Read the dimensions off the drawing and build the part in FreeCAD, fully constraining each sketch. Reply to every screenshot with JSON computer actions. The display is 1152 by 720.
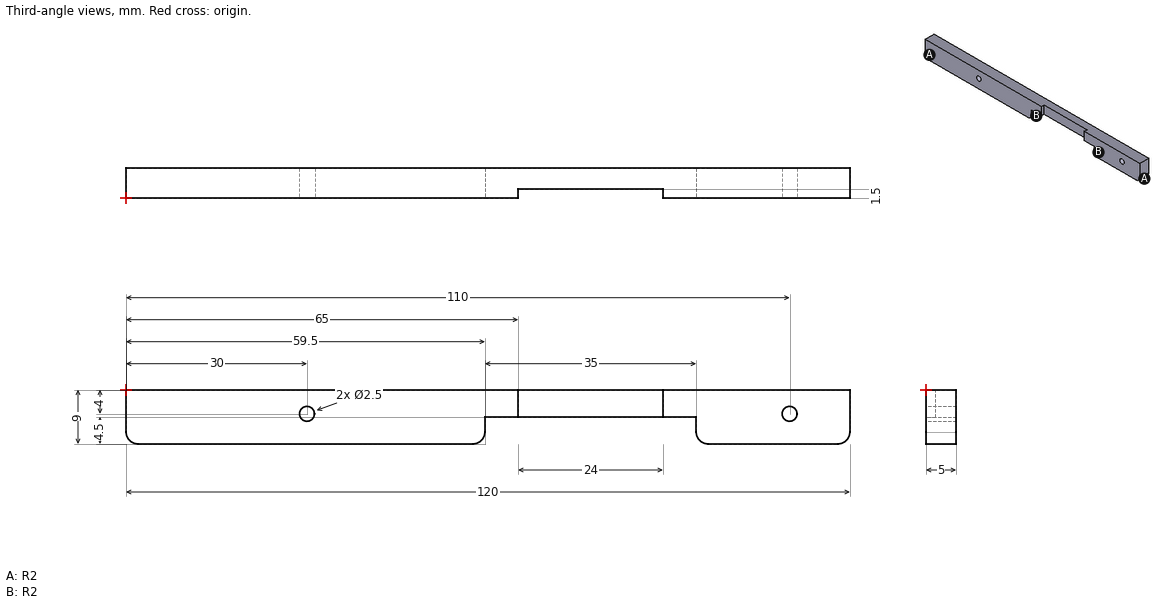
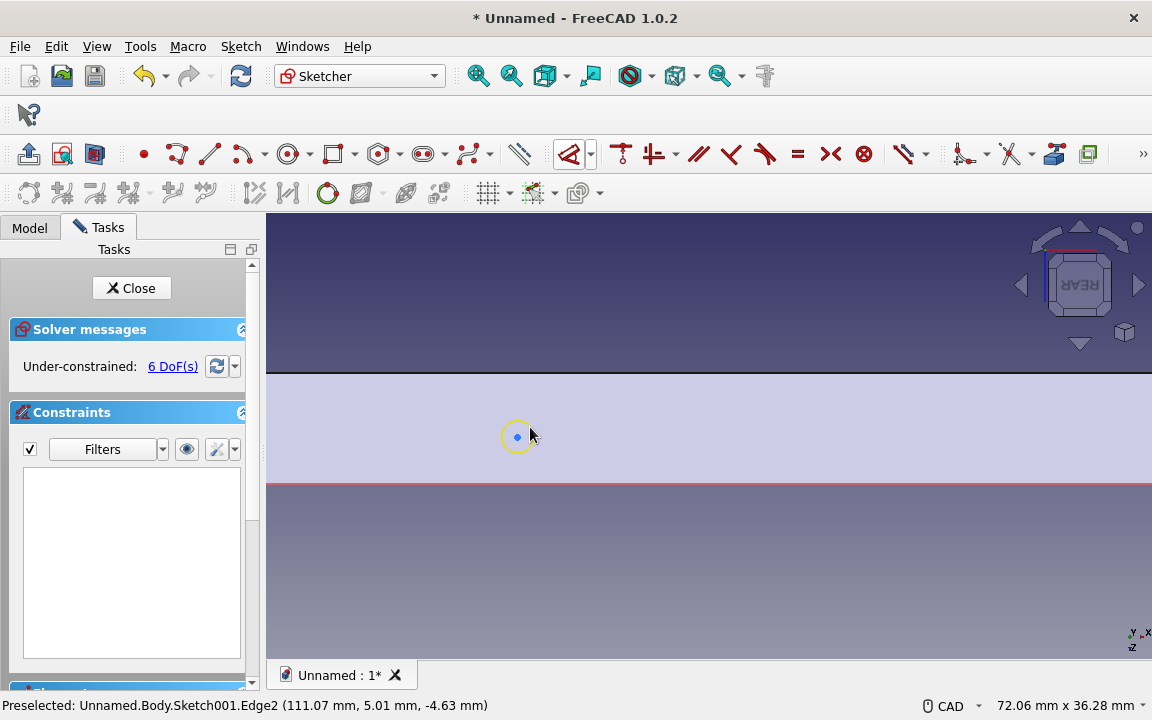
{"action": "left_click", "coordinate": [529, 426]}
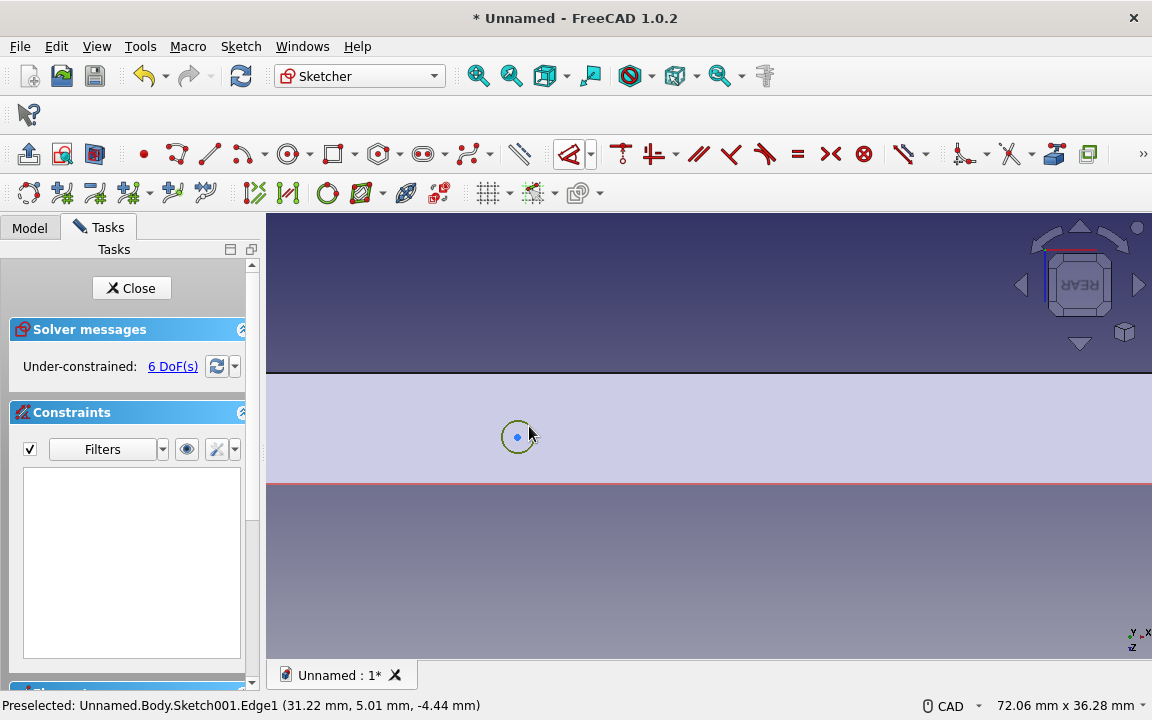
{"action": "scroll", "coordinate": [529, 427], "scroll_direction": "down", "scroll_amount": 5}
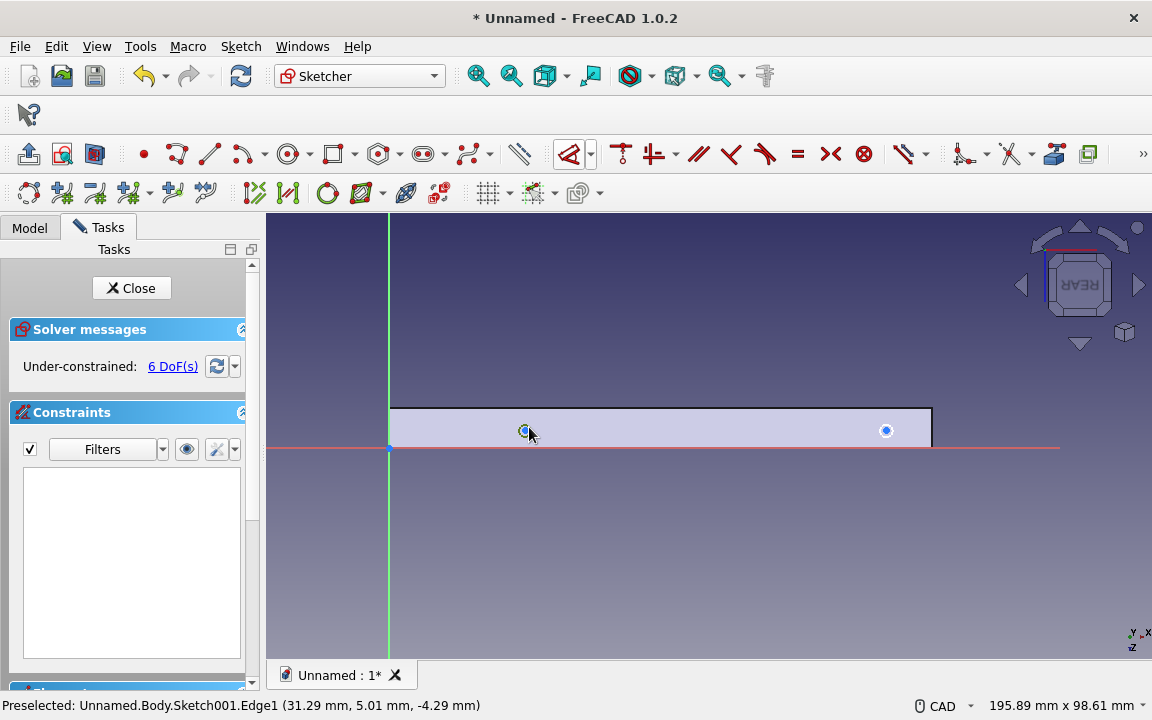
{"action": "scroll", "coordinate": [891, 427], "scroll_direction": "up", "scroll_amount": 4}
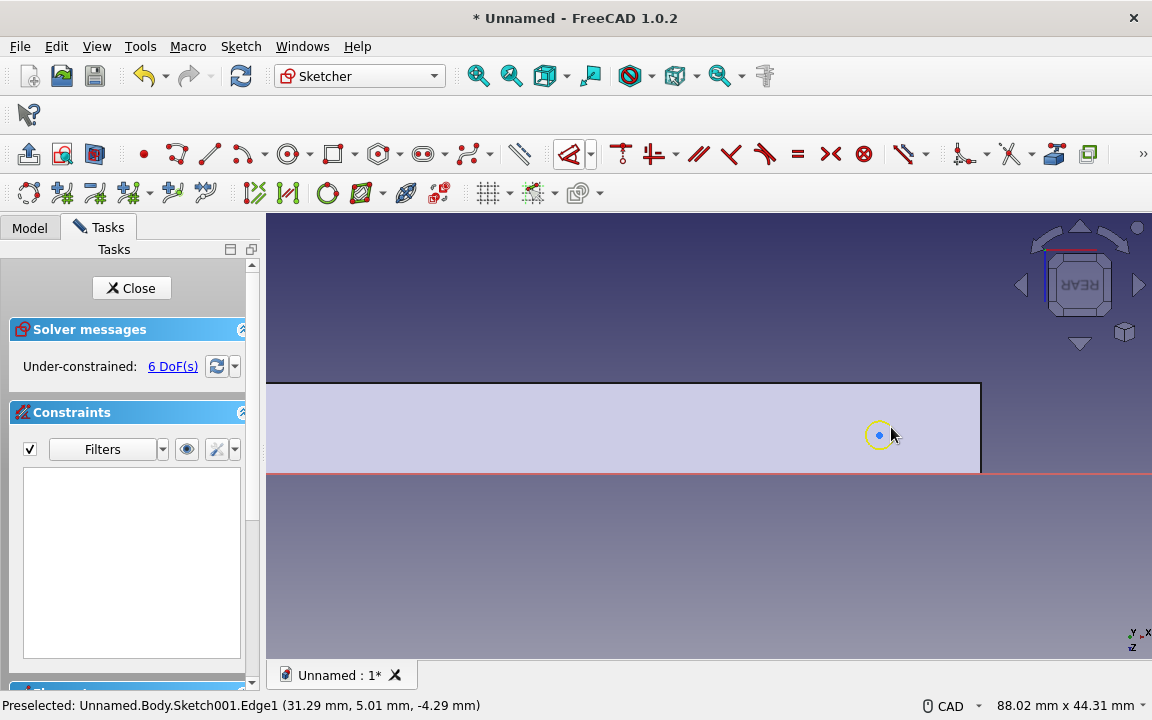
{"action": "left_click", "coordinate": [890, 425]}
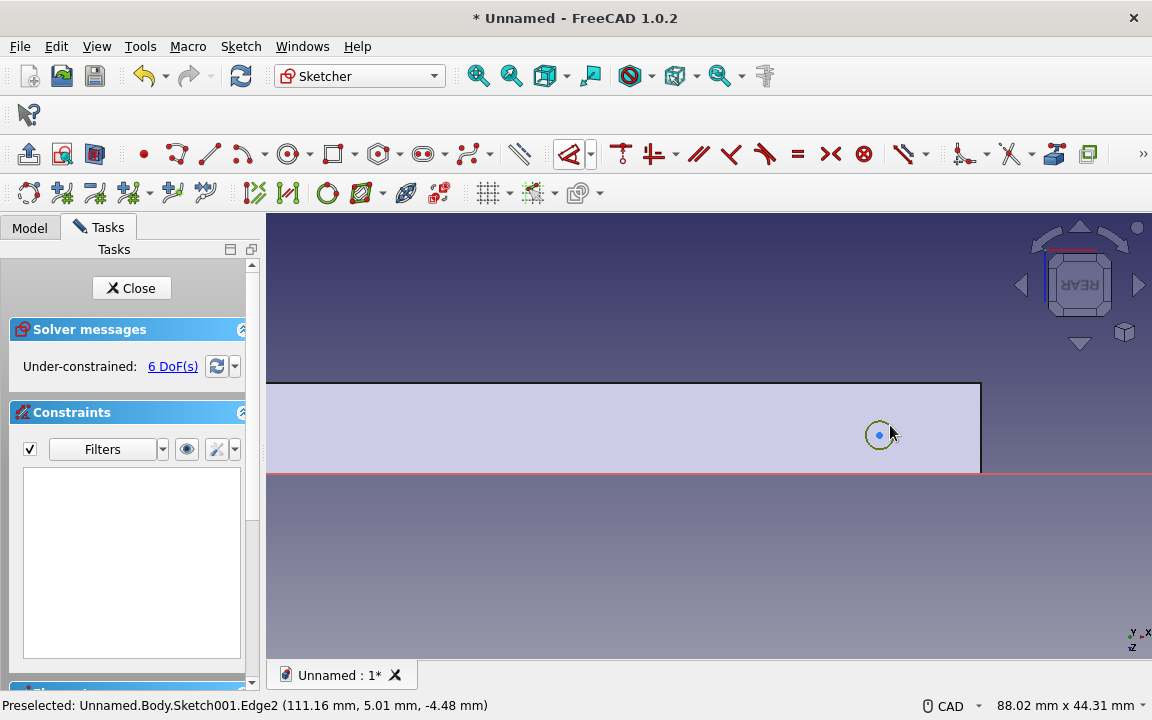
{"action": "key", "text": "e"}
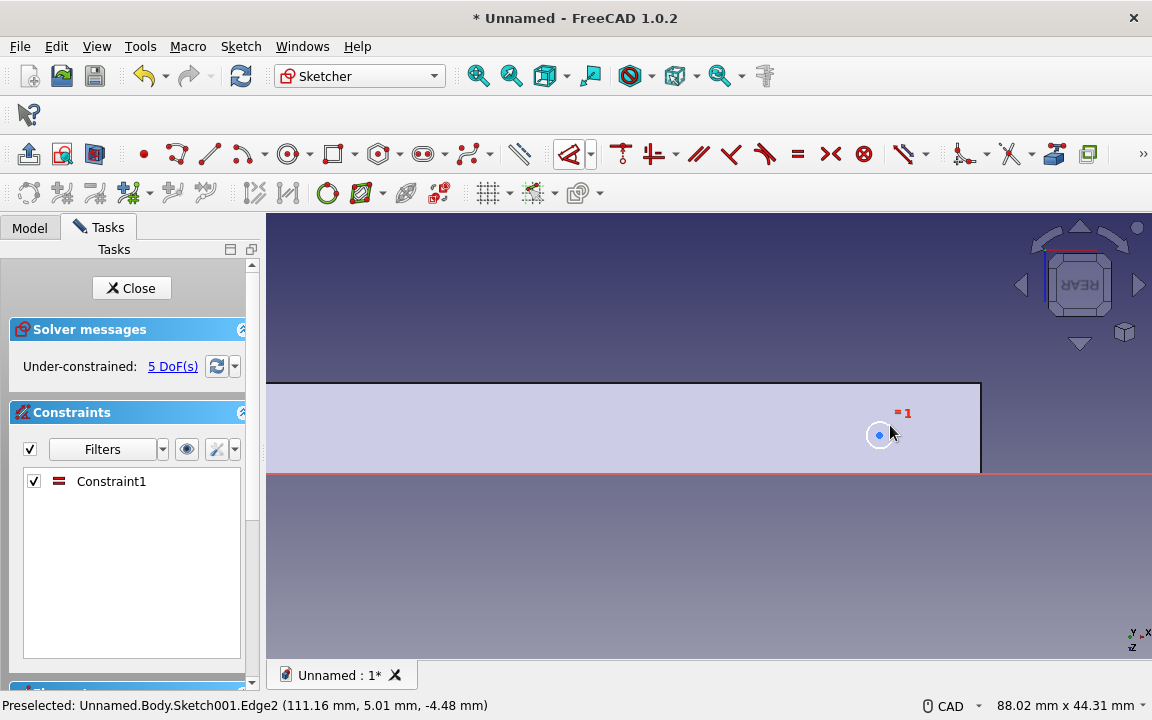
{"action": "key", "text": "d"}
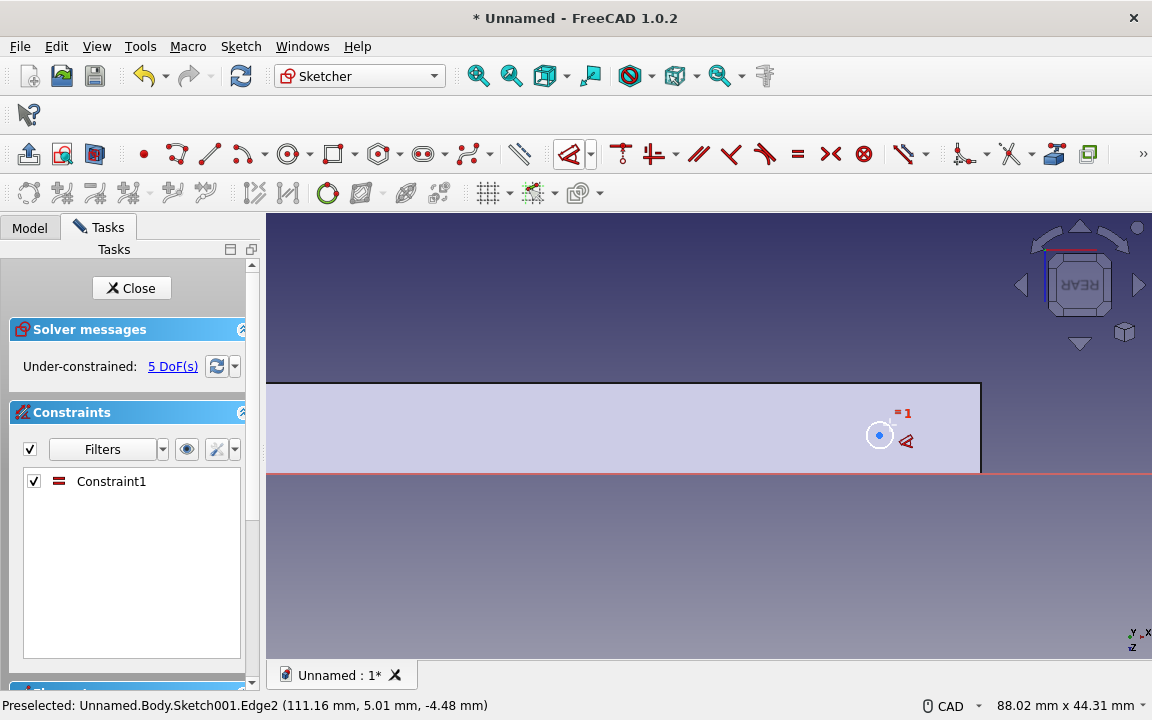
{"action": "scroll", "coordinate": [891, 427], "scroll_direction": "down", "scroll_amount": 4}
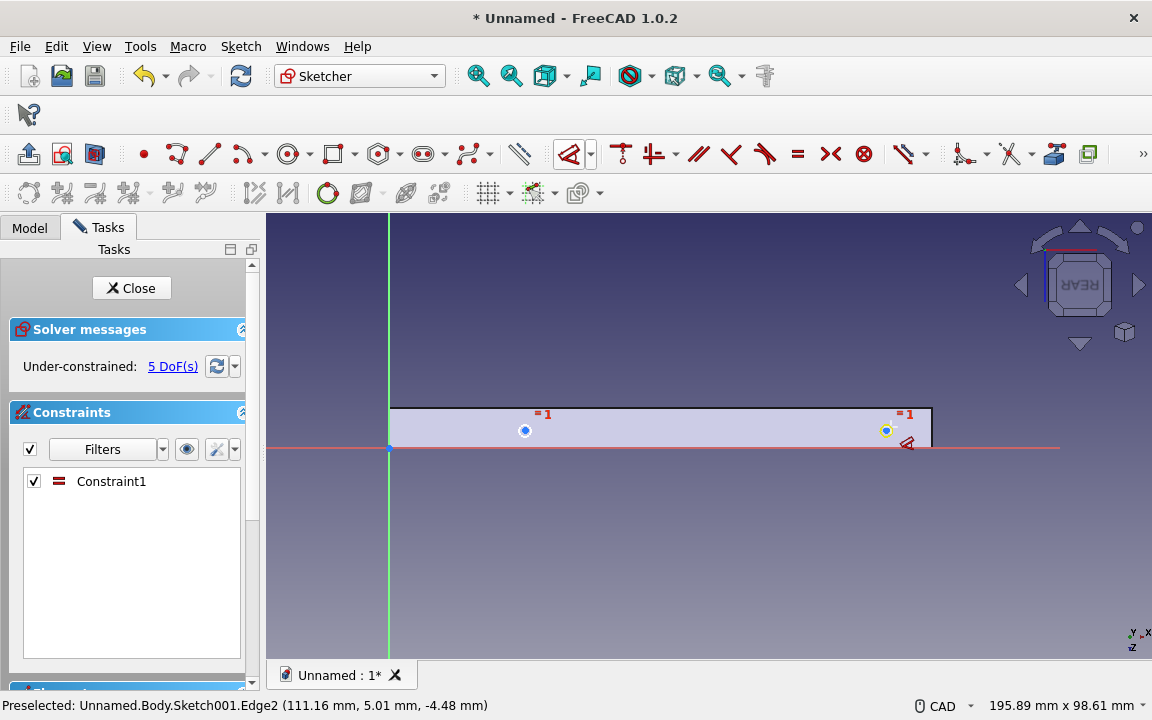
{"action": "scroll", "coordinate": [529, 427], "scroll_direction": "up", "scroll_amount": 7}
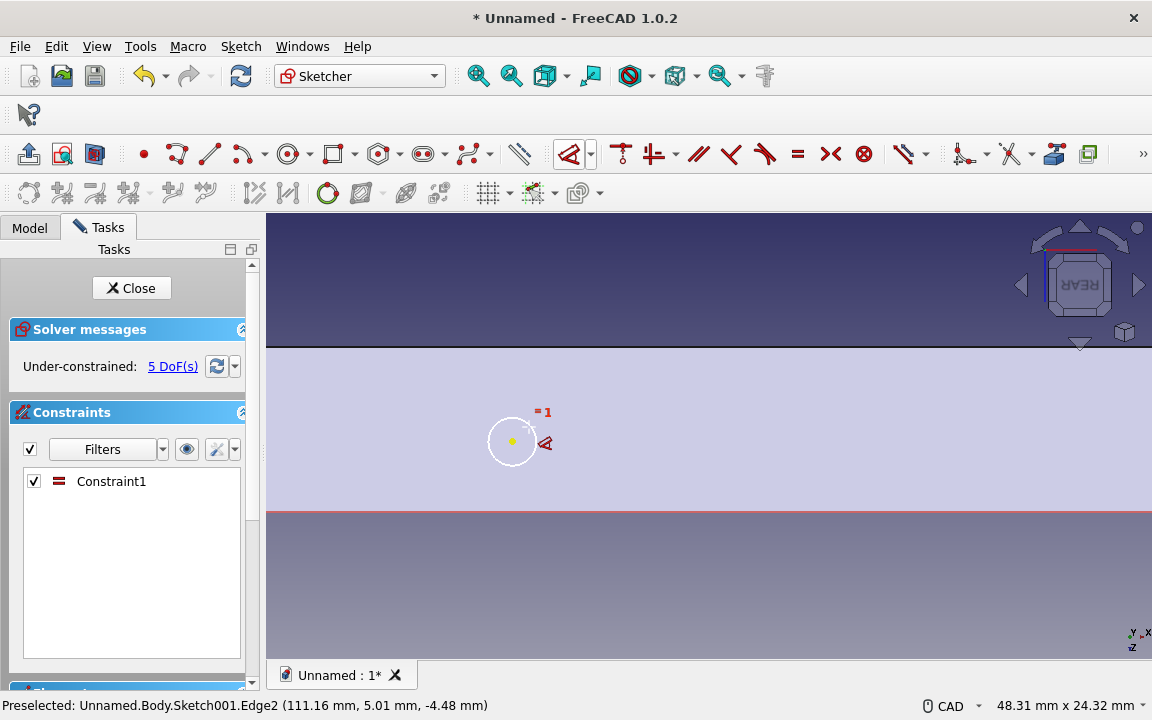
{"action": "left_click", "coordinate": [529, 425]}
{"action": "left_click", "coordinate": [552, 402]}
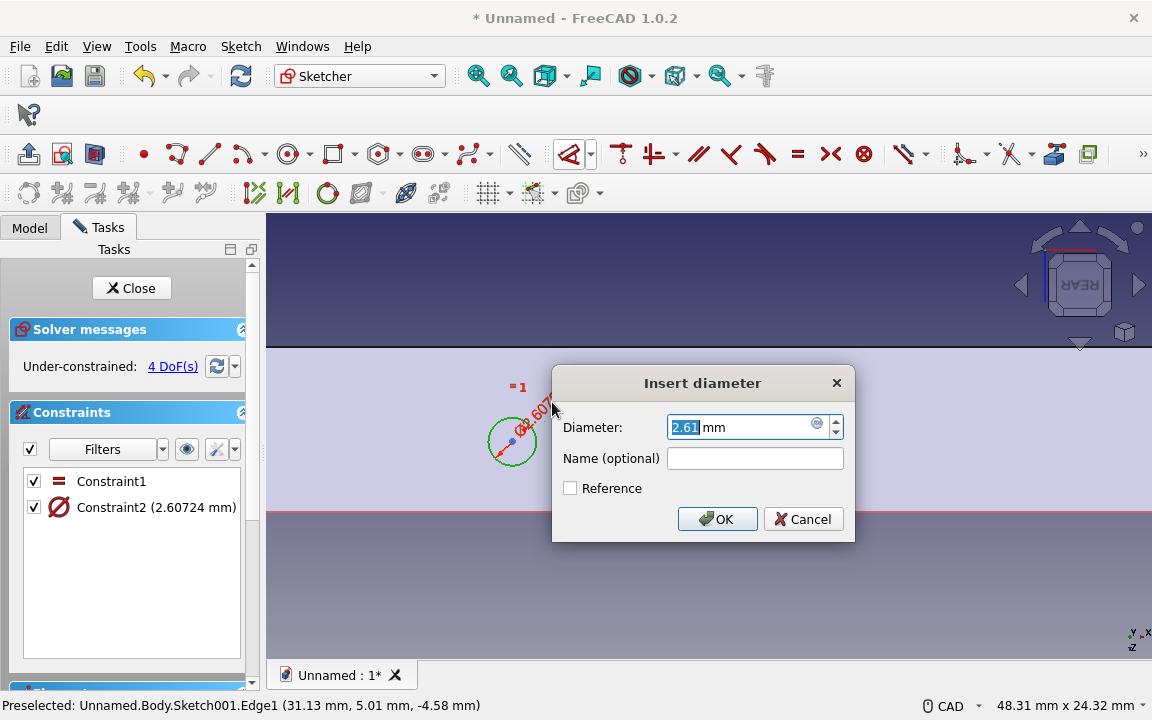
{"action": "type", "text": "2.5"}
{"action": "key", "text": "Return"}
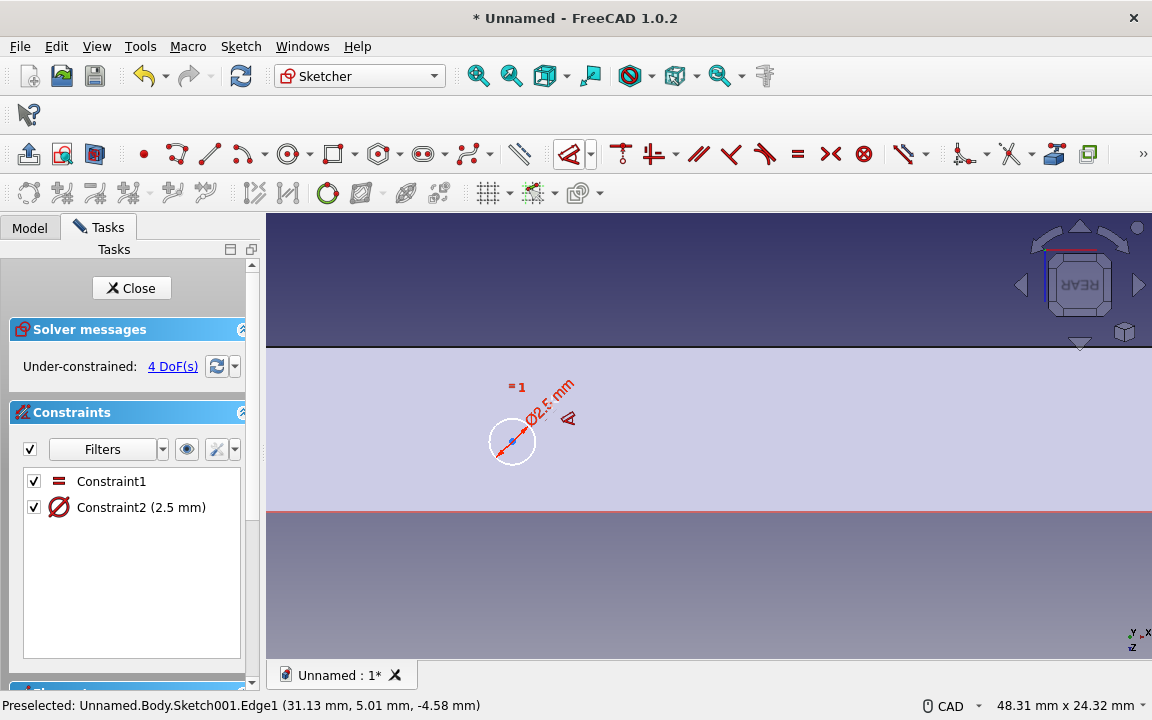
{"action": "left_click", "coordinate": [512, 442]}
{"action": "left_click", "coordinate": [546, 477]}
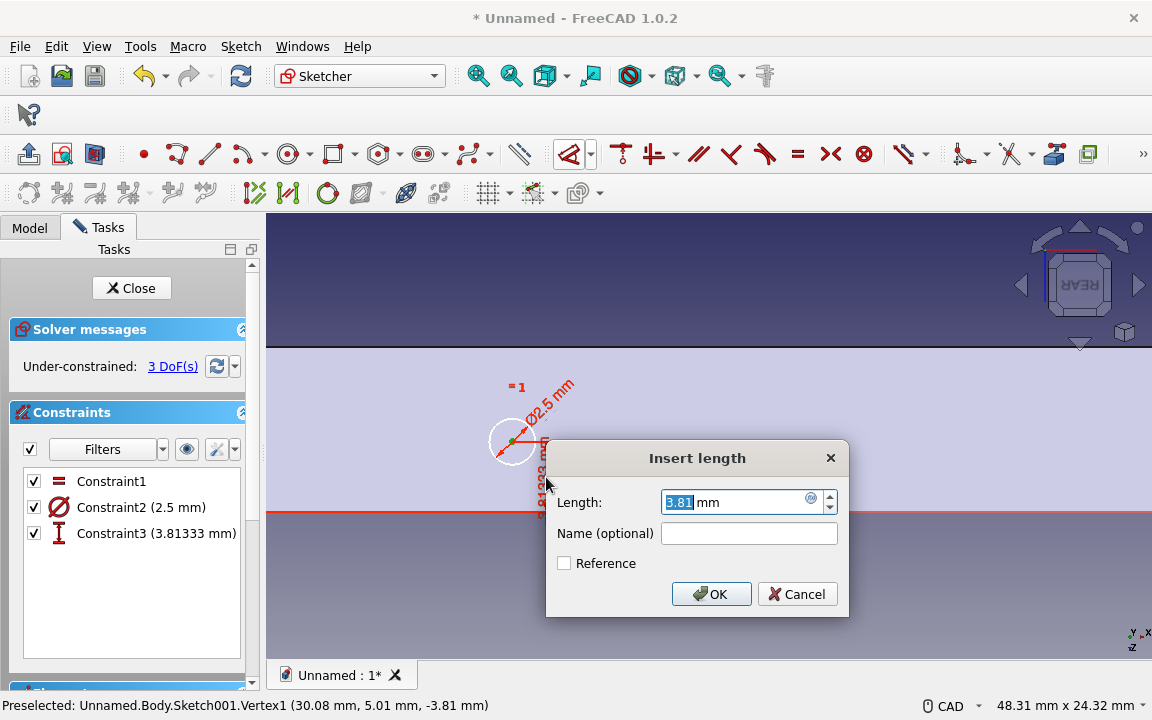
{"action": "type", "text": "4"}
{"action": "key", "text": "Return"}